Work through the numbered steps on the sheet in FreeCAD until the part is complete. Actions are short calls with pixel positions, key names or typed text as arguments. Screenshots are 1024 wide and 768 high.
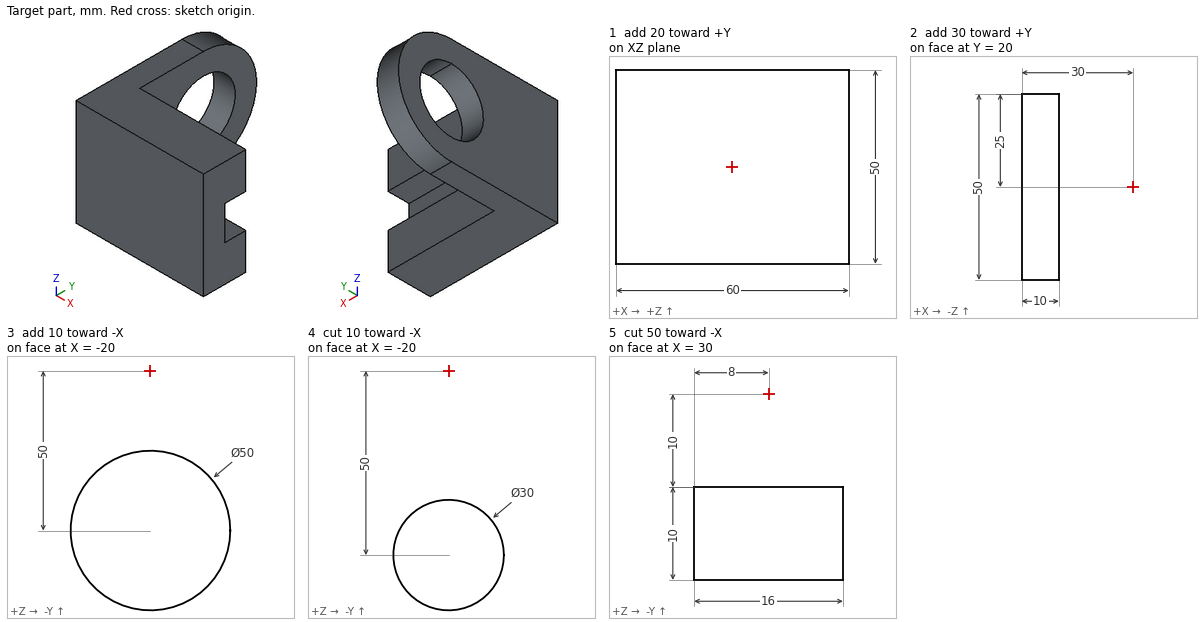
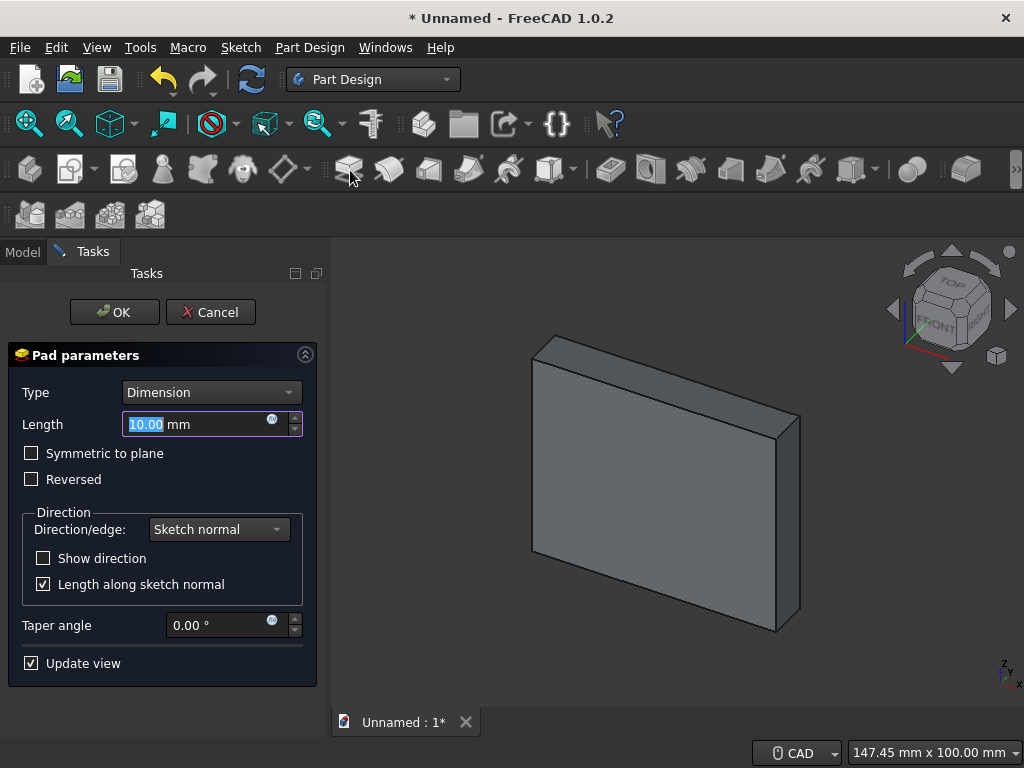
text(20)
key(Tab)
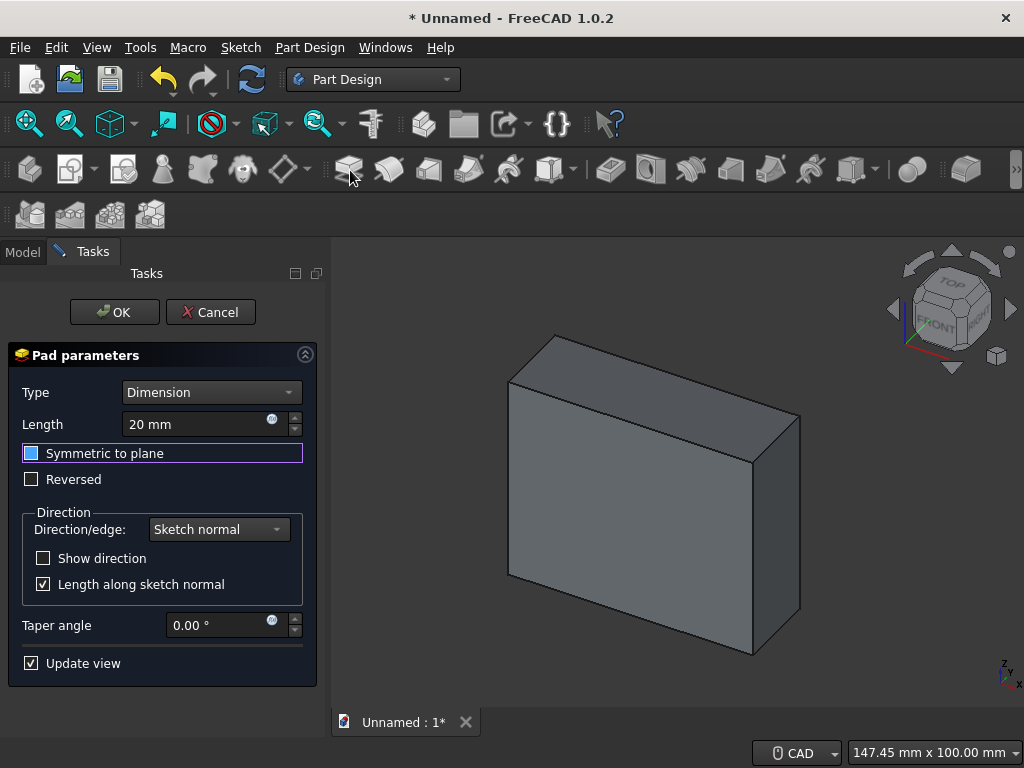
click(30, 479)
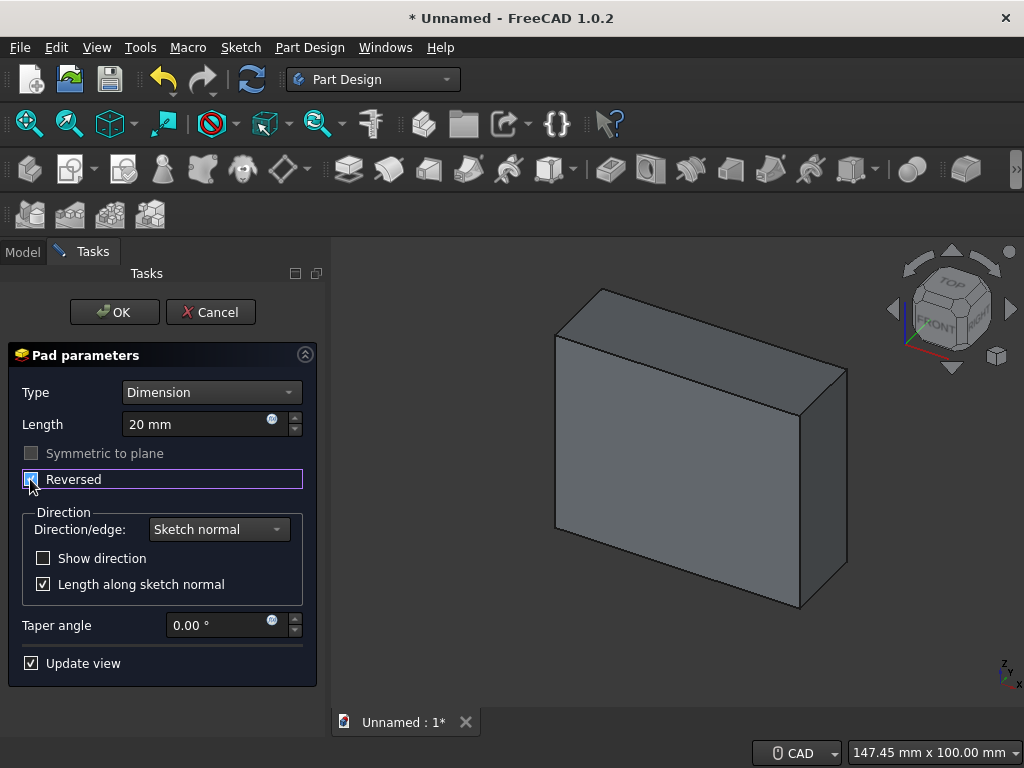
click(115, 312)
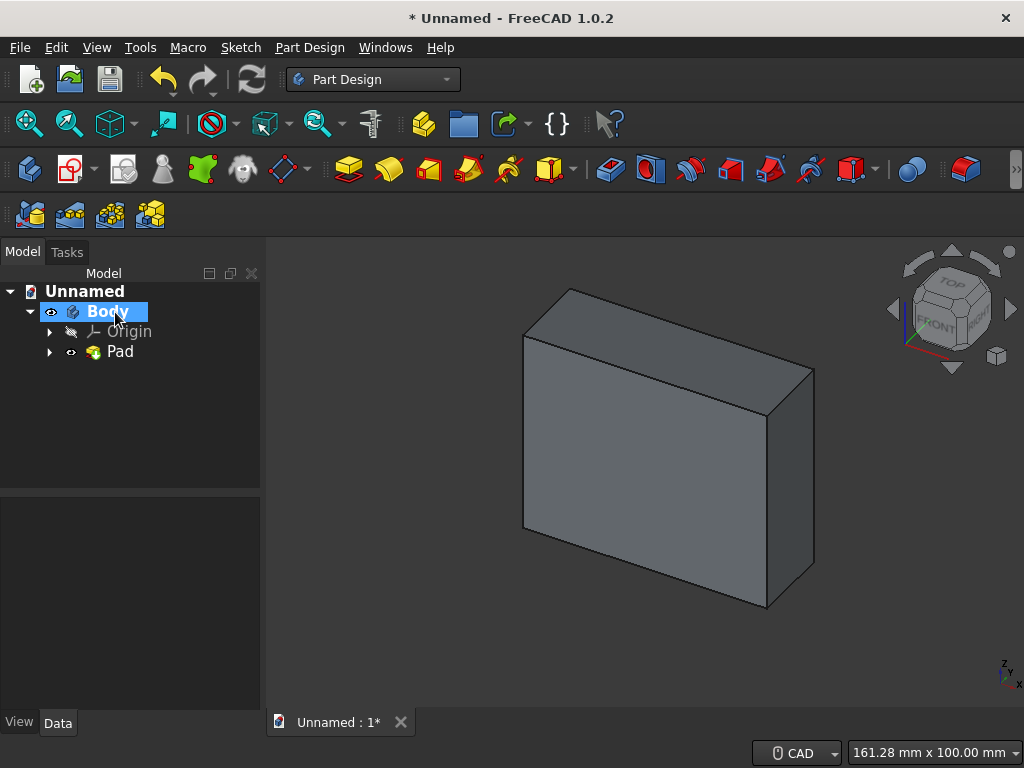
key(4)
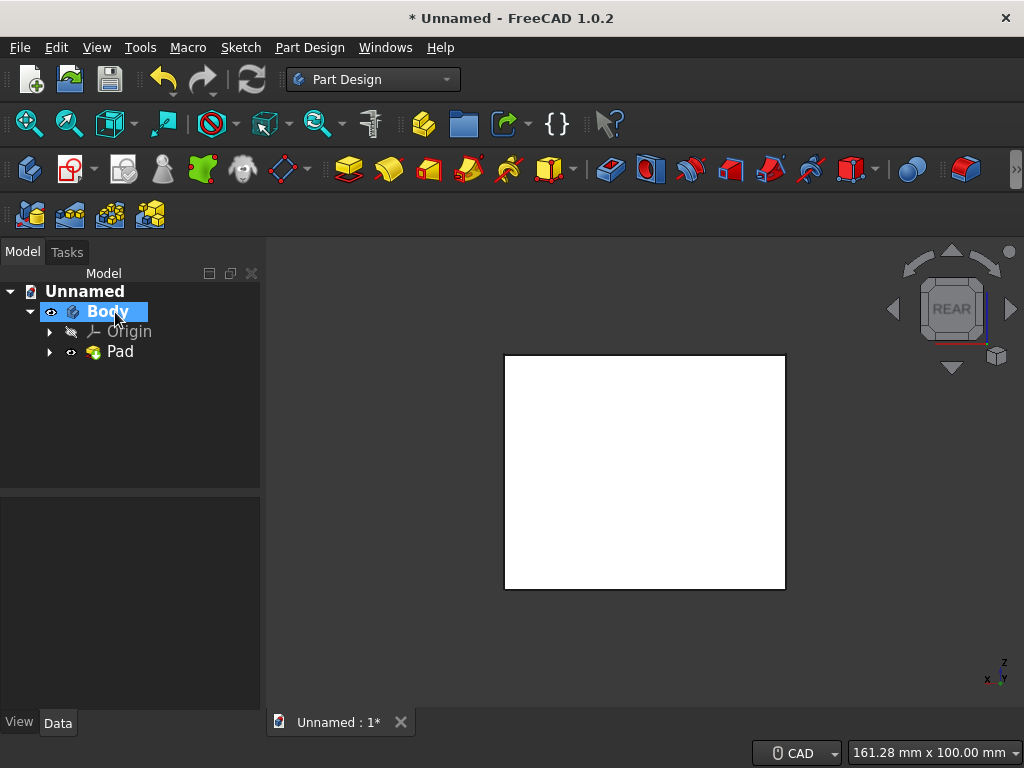
click(645, 471)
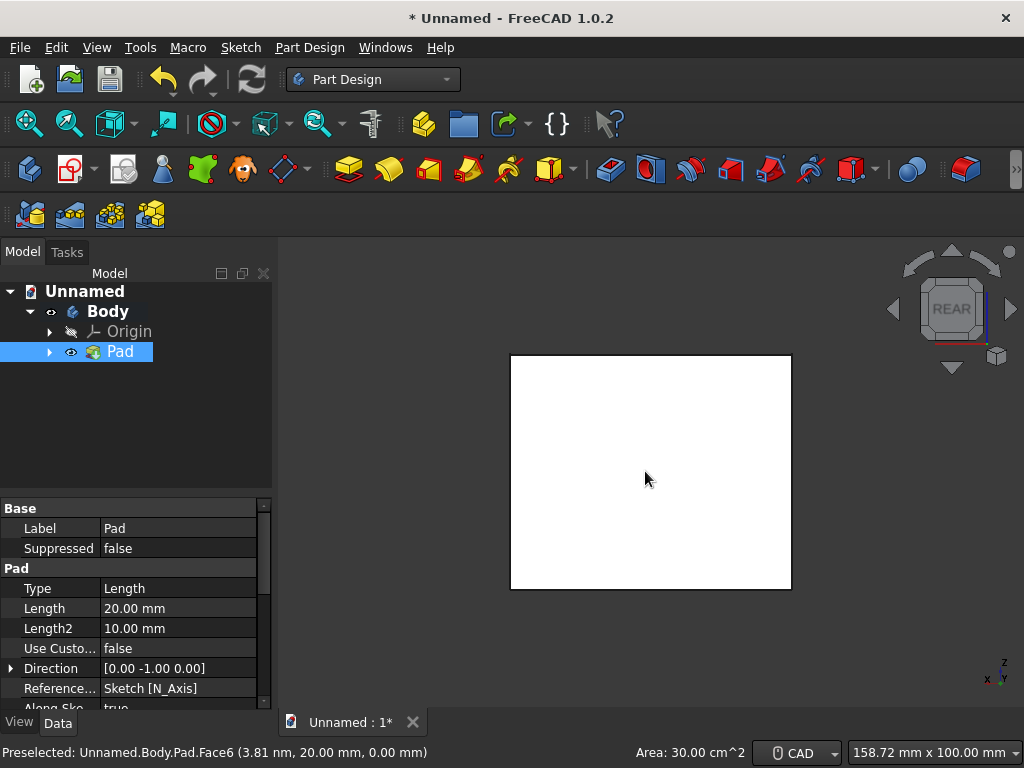
click(70, 170)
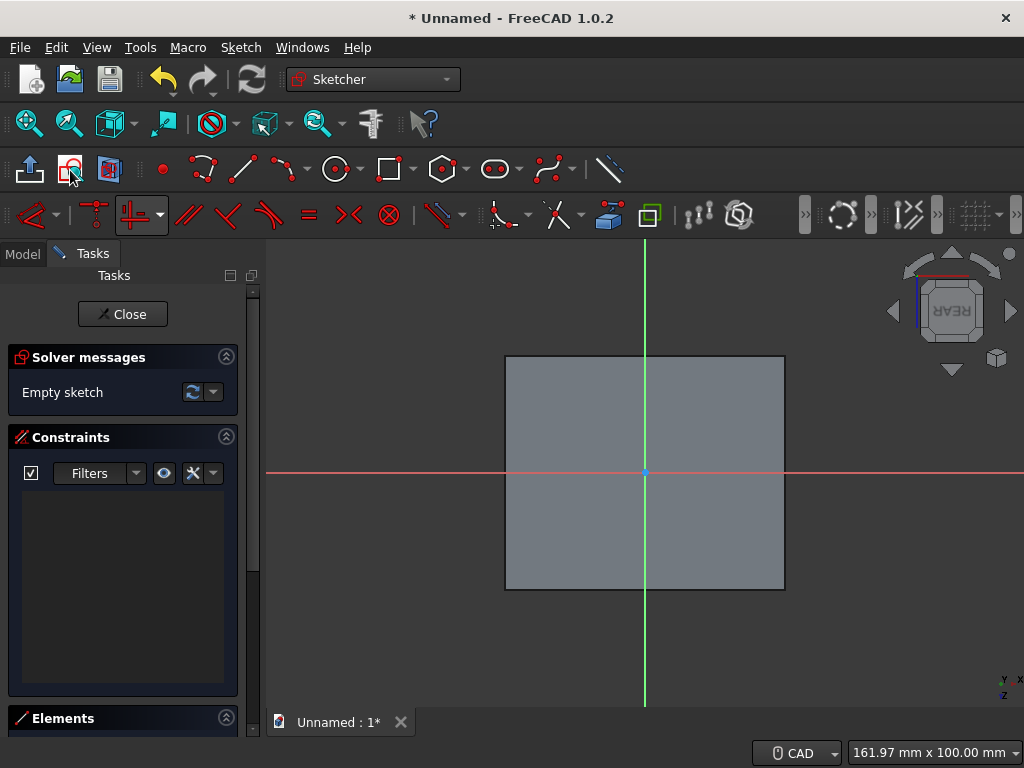
click(390, 170)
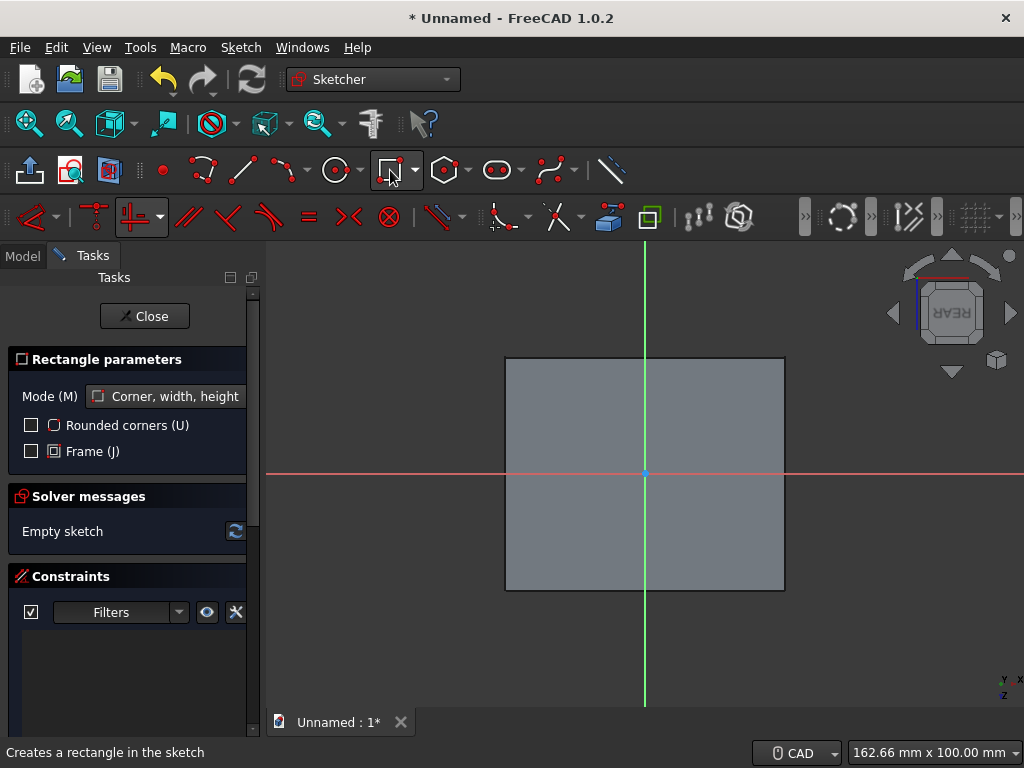
click(505, 358)
click(552, 591)
key(Escape)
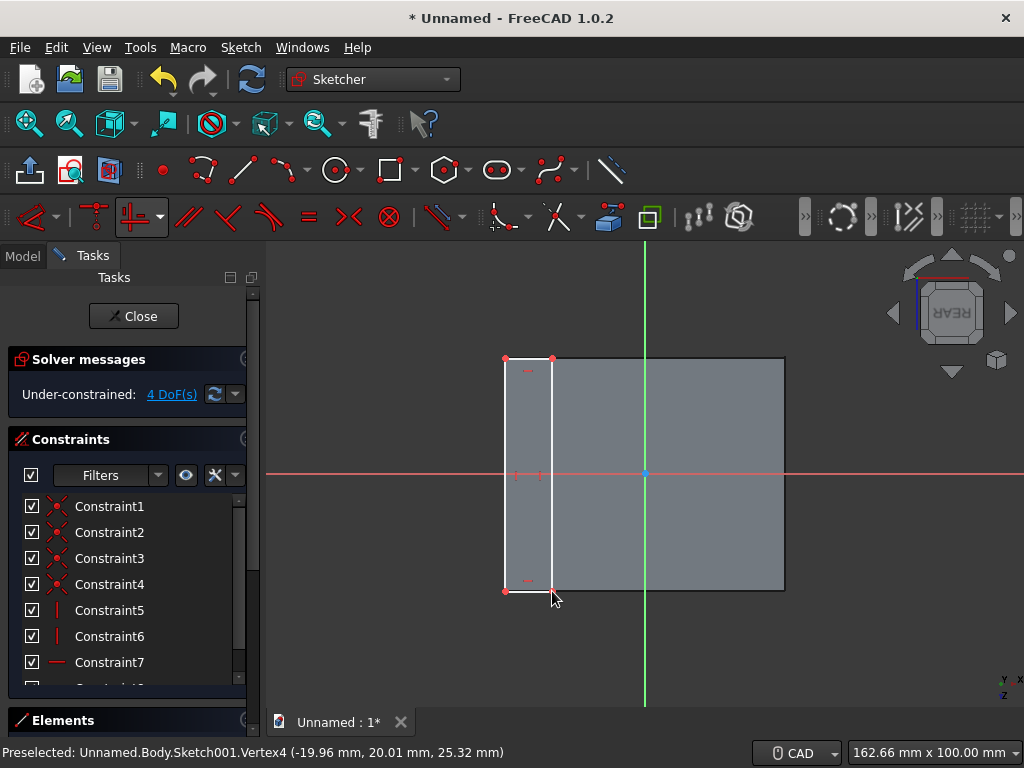
click(32, 218)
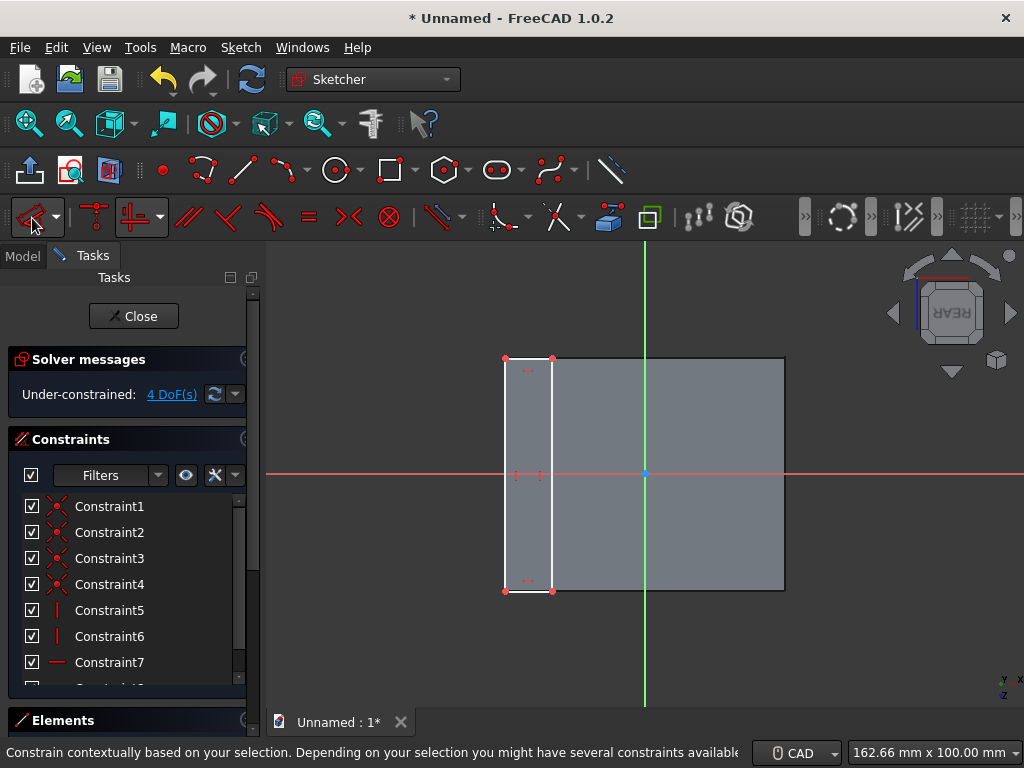
click(505, 429)
click(471, 422)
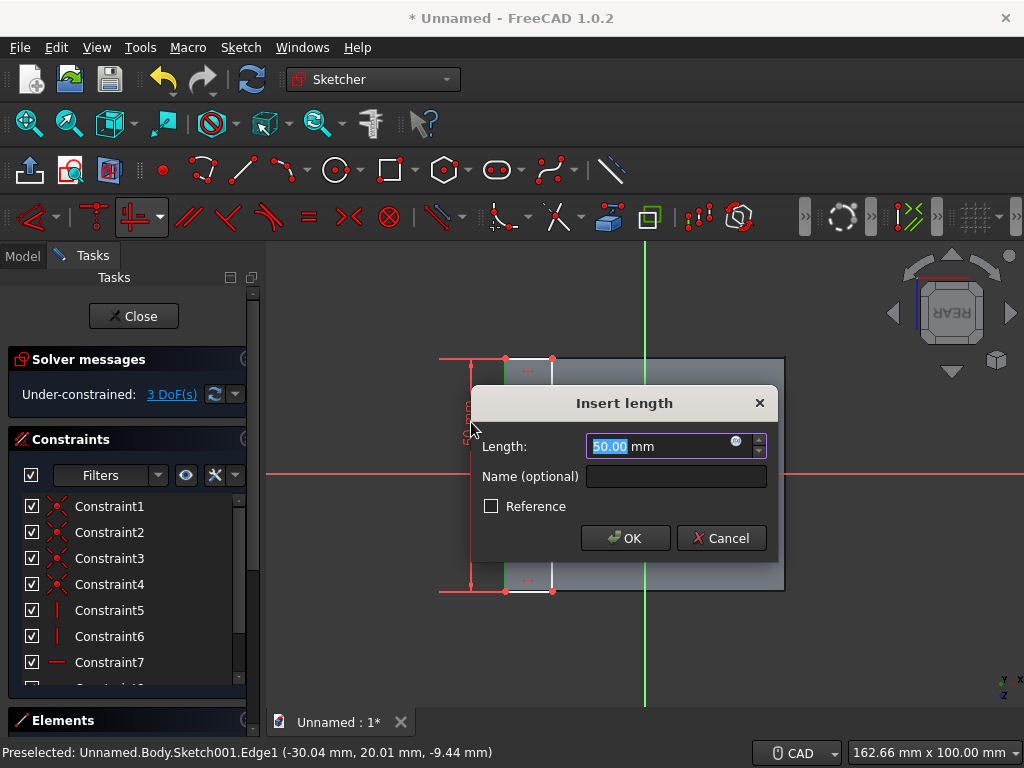
text(50)
key(Return)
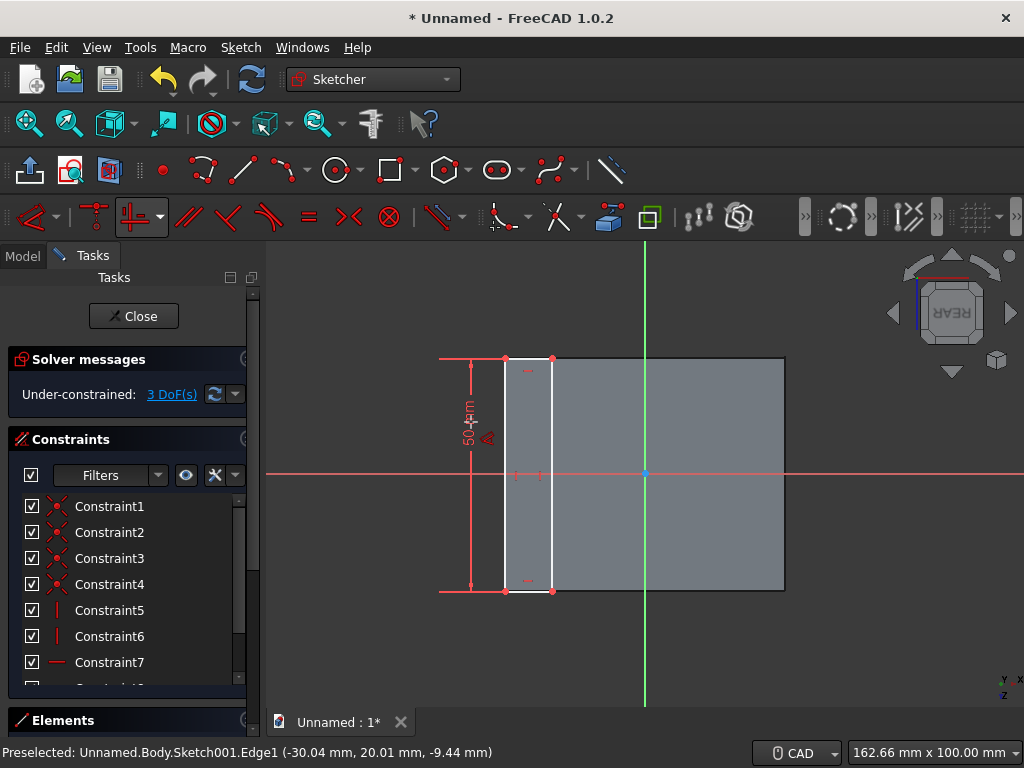
click(519, 592)
click(529, 626)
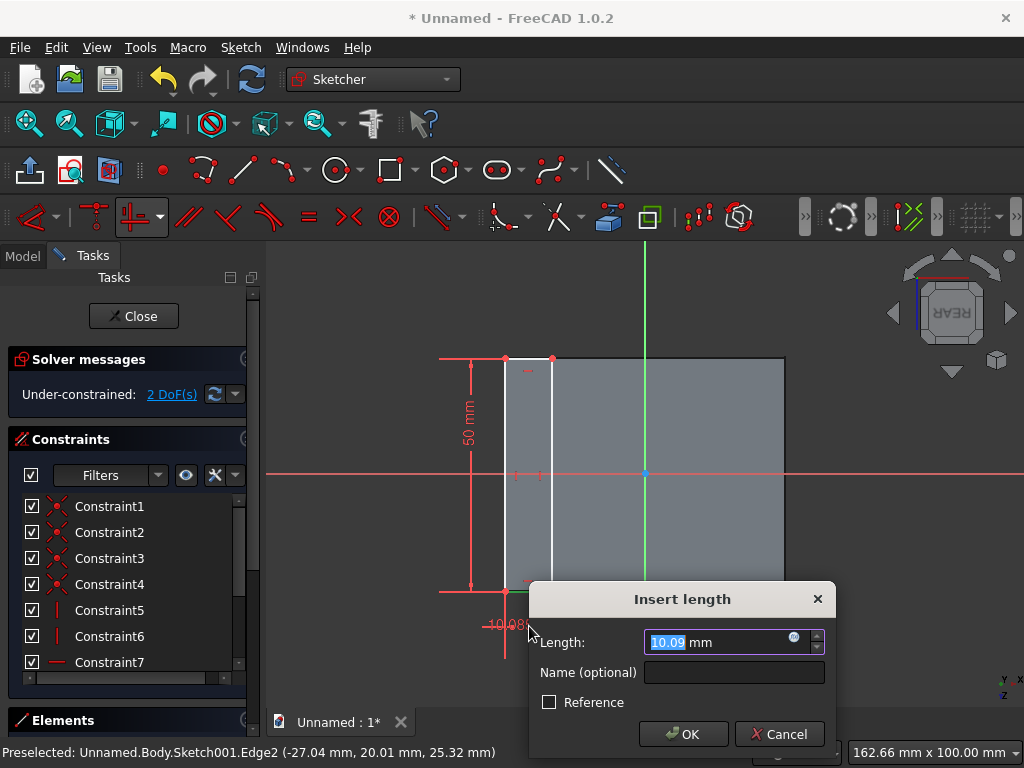
text(10)
key(Return)